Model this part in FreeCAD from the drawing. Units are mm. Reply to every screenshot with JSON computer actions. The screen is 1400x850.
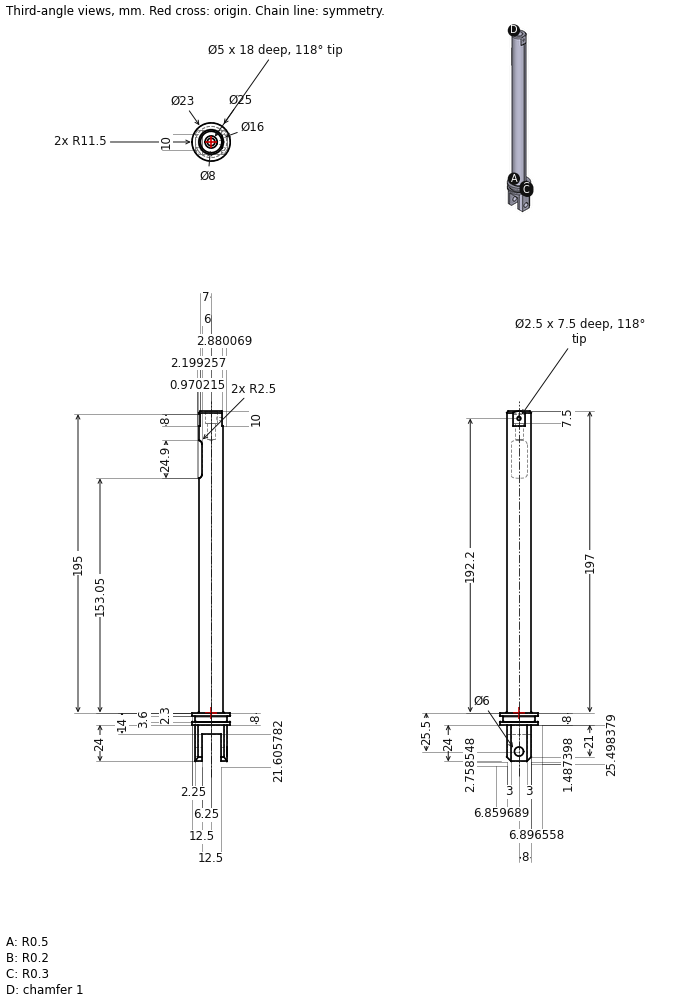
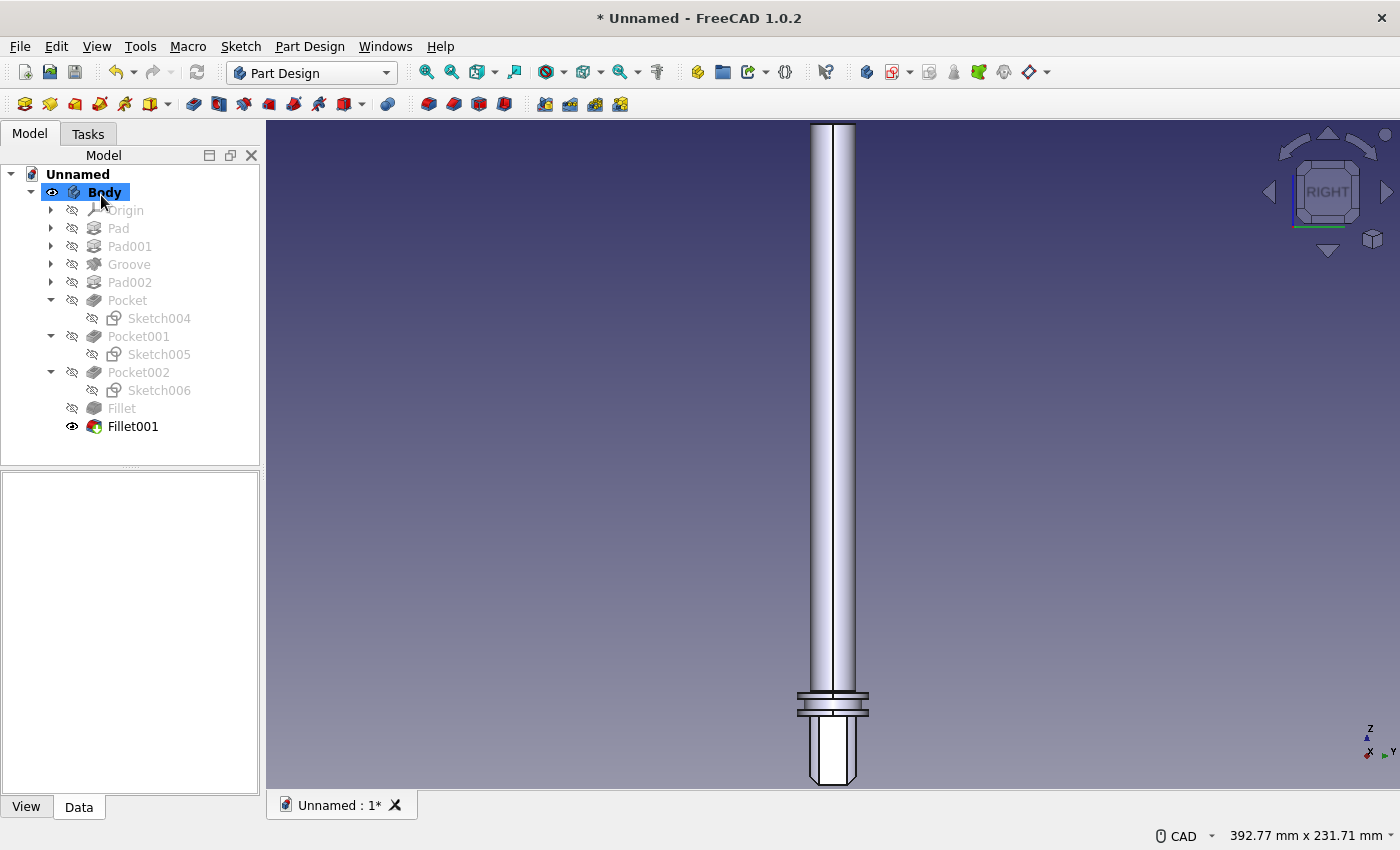
{"action": "key", "text": "0"}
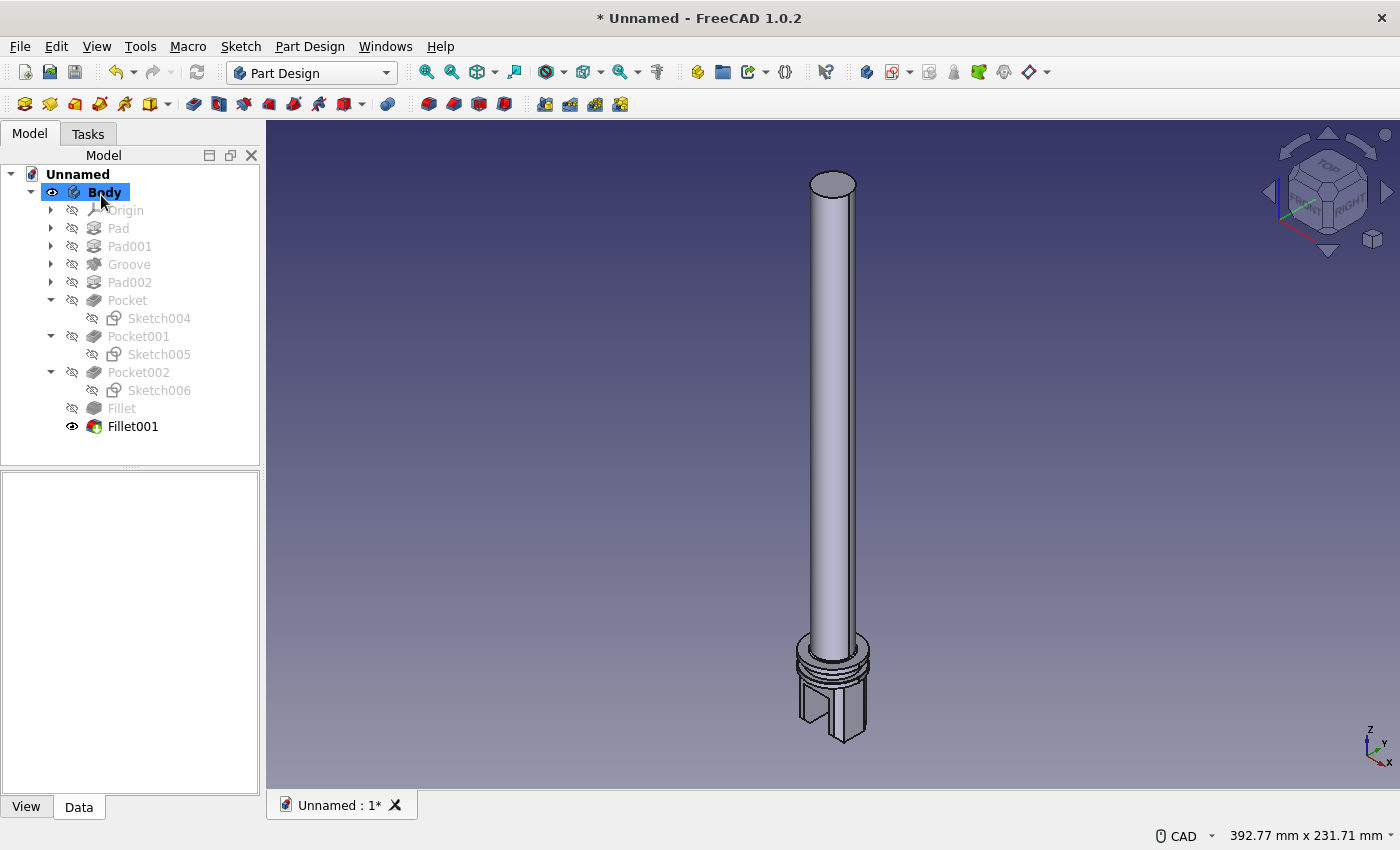
{"action": "key", "text": "2"}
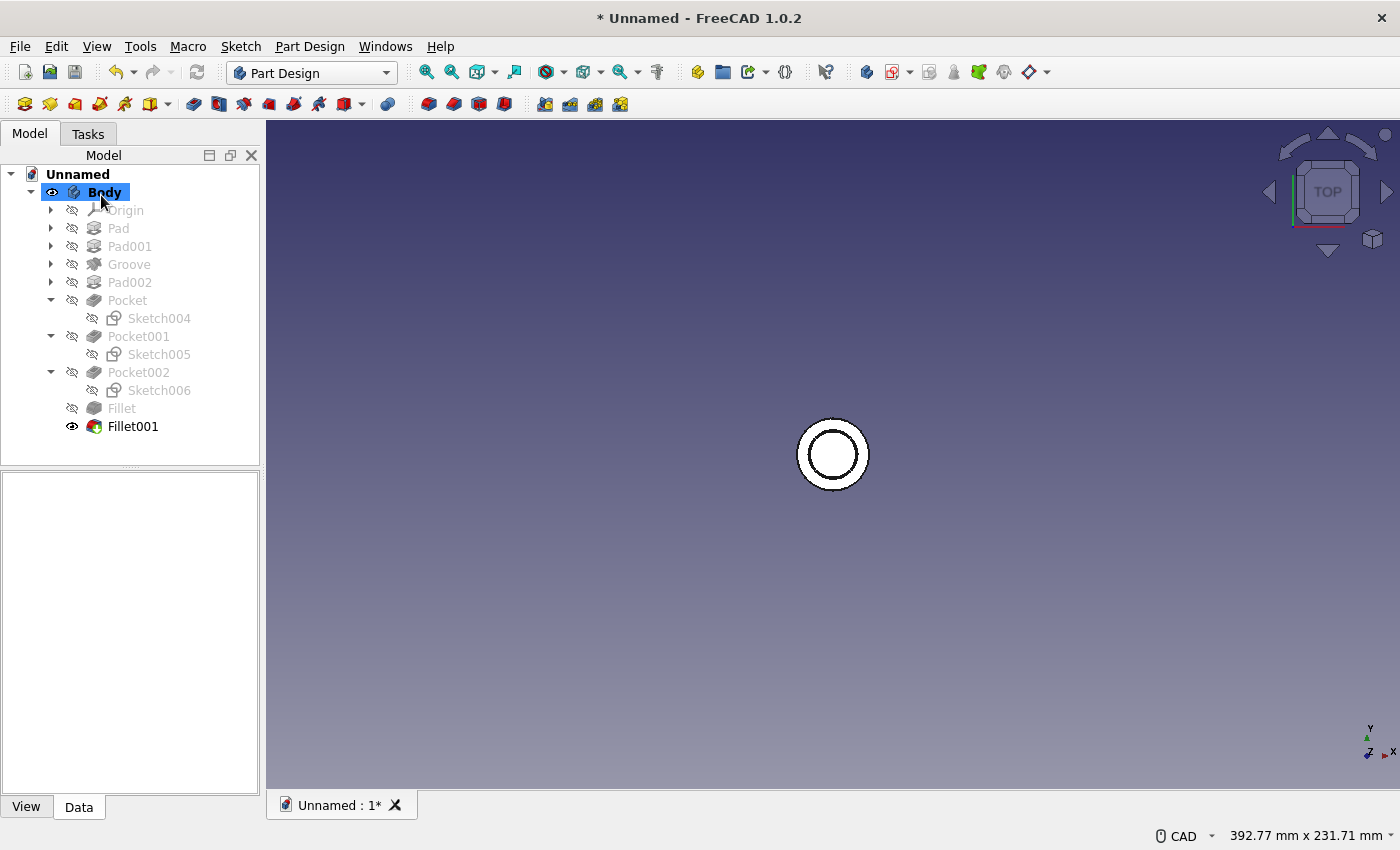
{"action": "left_click", "coordinate": [427, 72]}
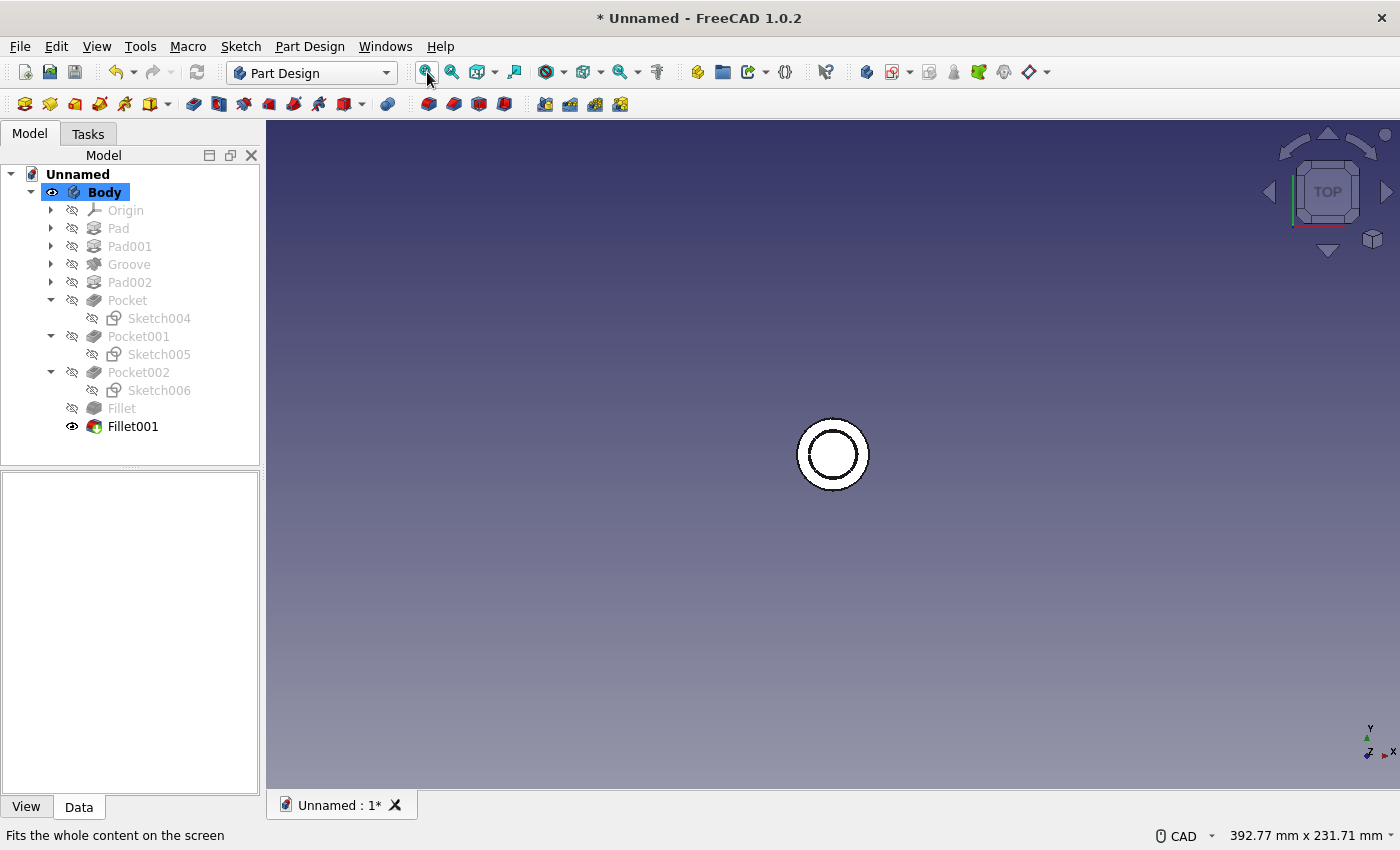
{"action": "key", "text": "1"}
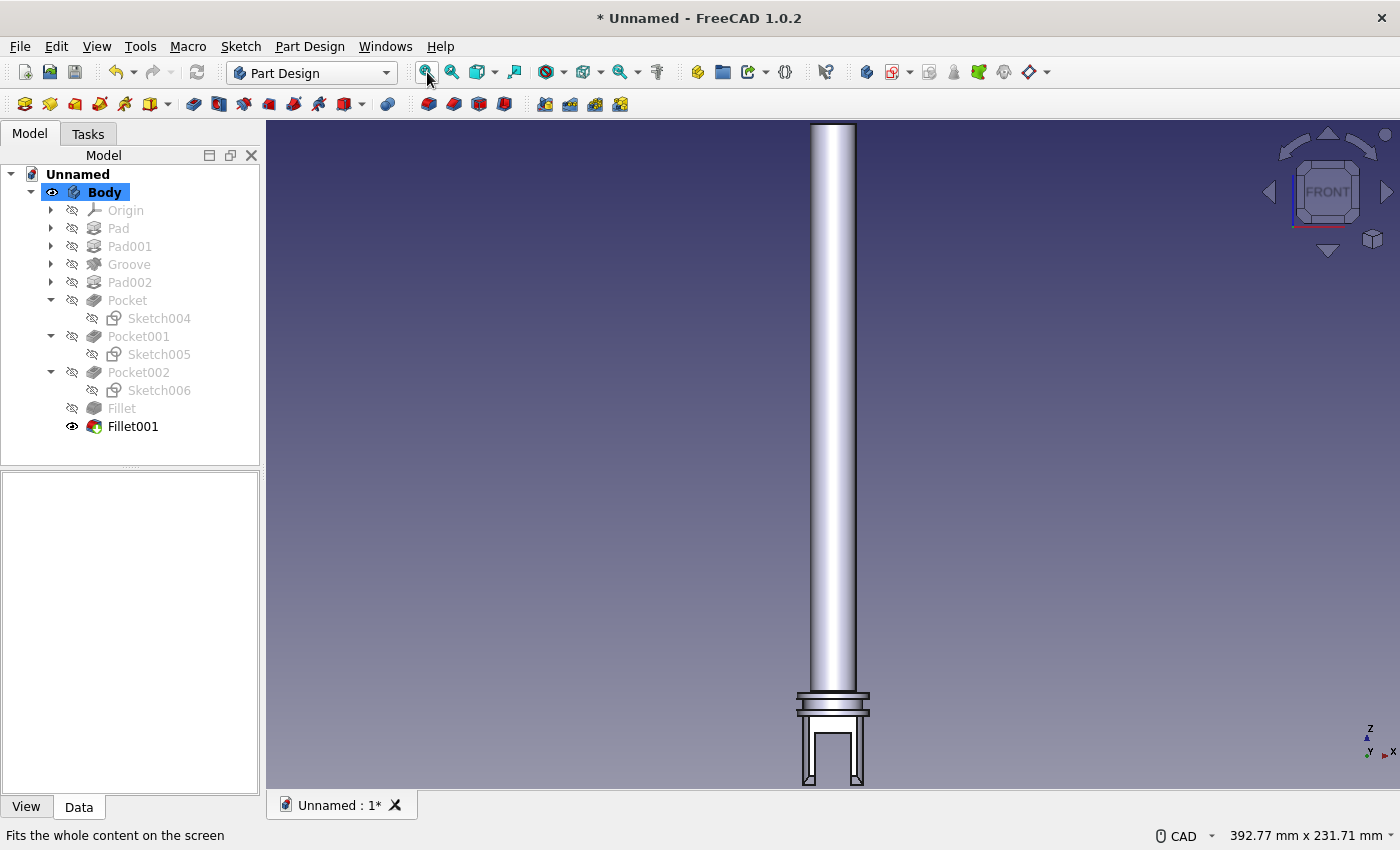
{"action": "key", "text": "3"}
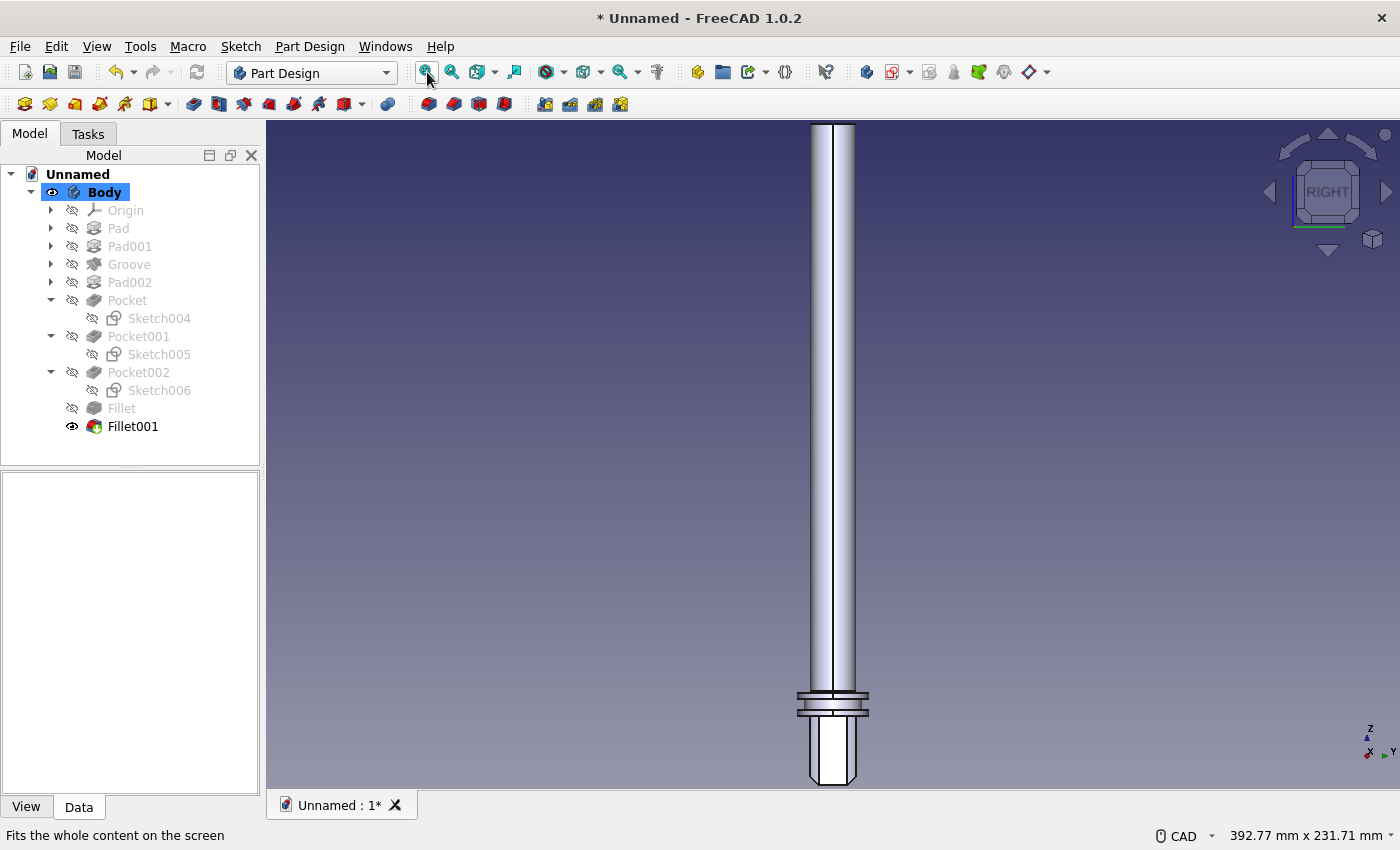
{"action": "key", "text": "5"}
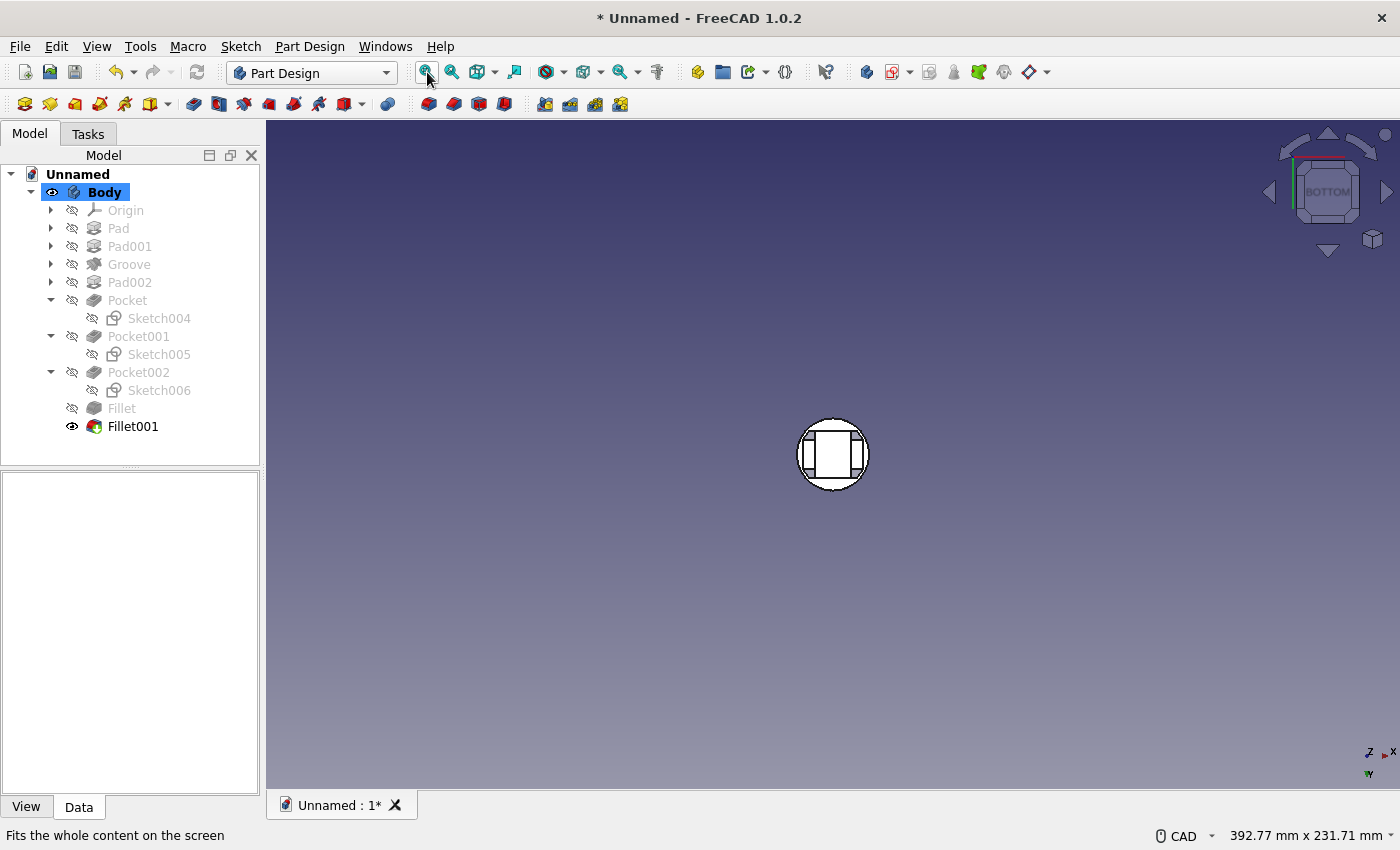
{"action": "left_click", "coordinate": [427, 72]}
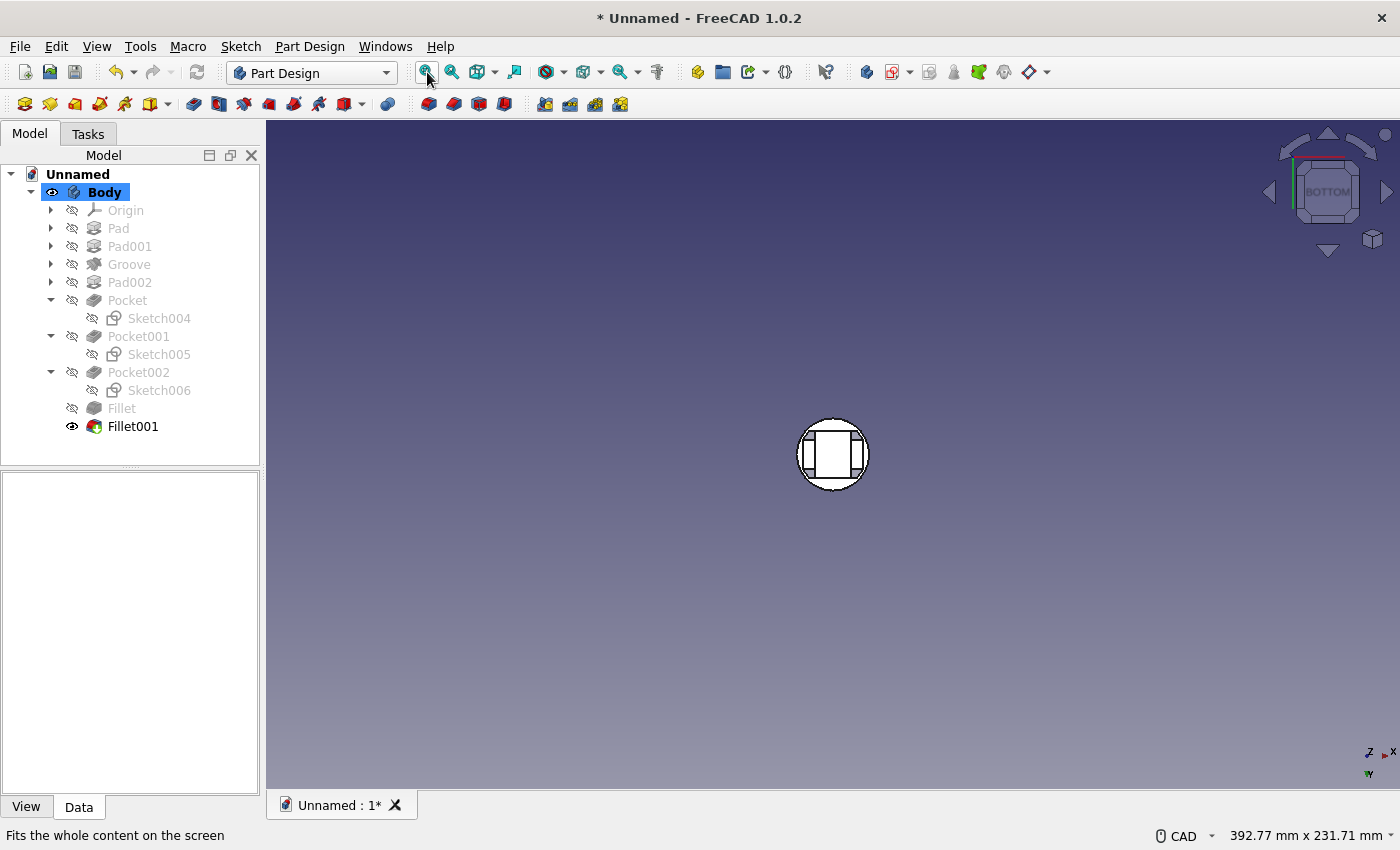
{"action": "key", "text": "4"}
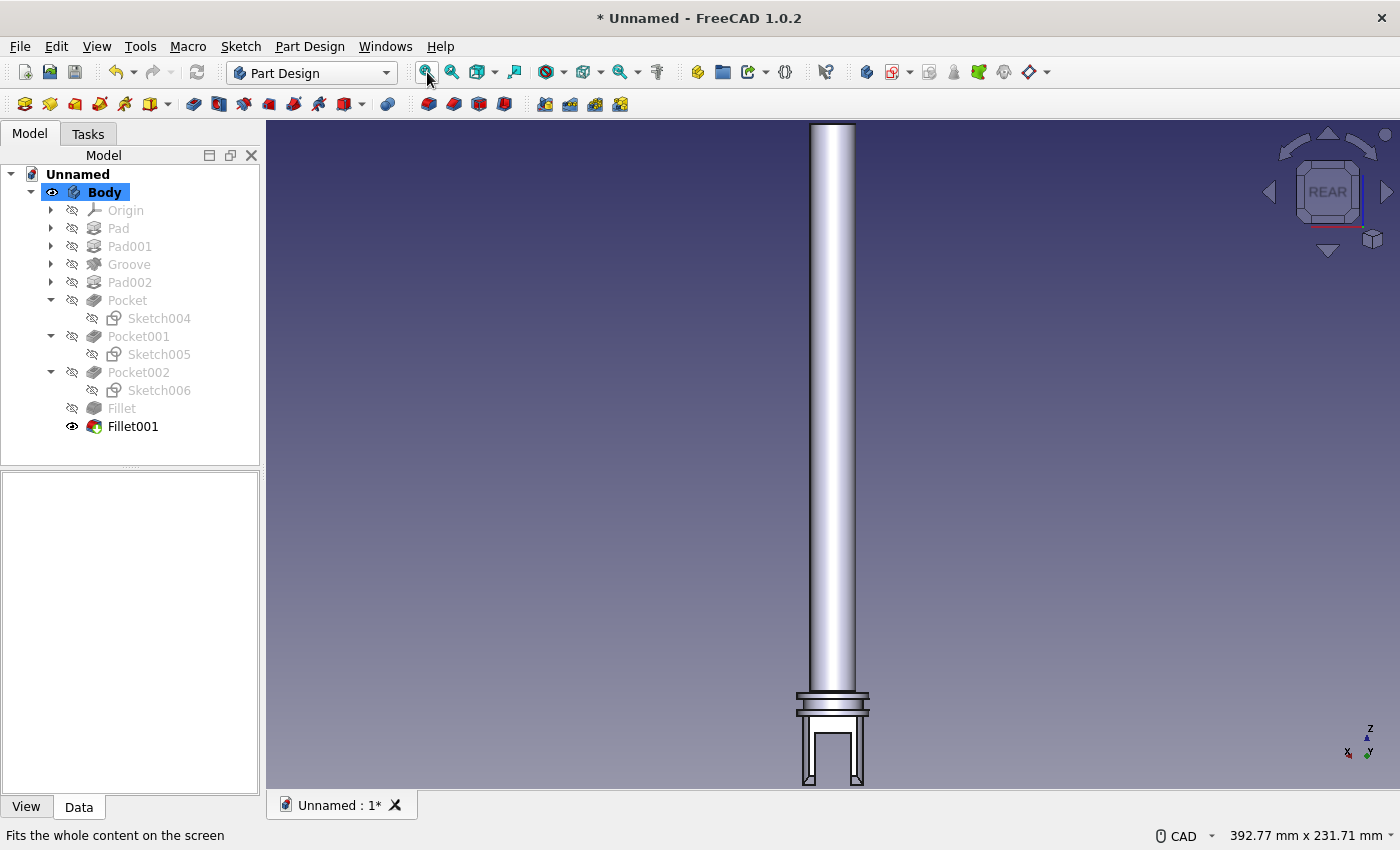
{"action": "key", "text": "6"}